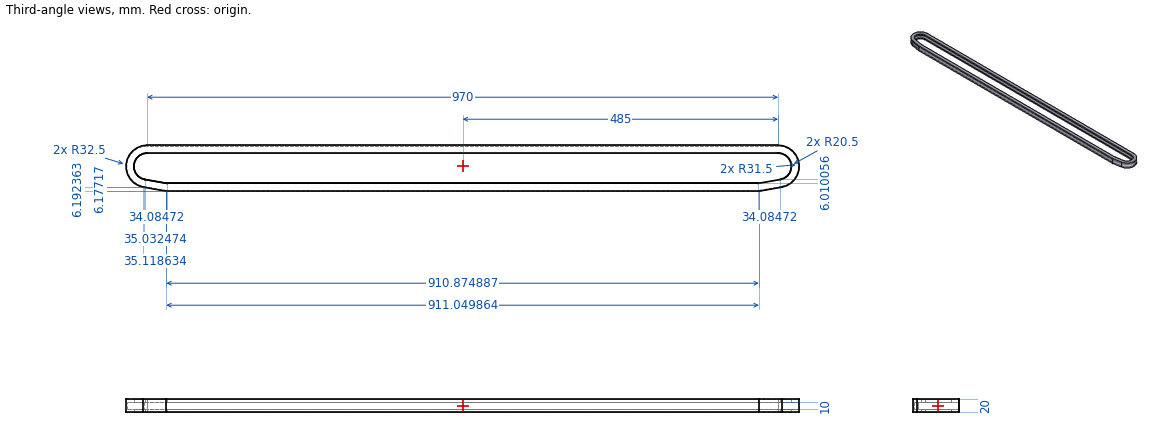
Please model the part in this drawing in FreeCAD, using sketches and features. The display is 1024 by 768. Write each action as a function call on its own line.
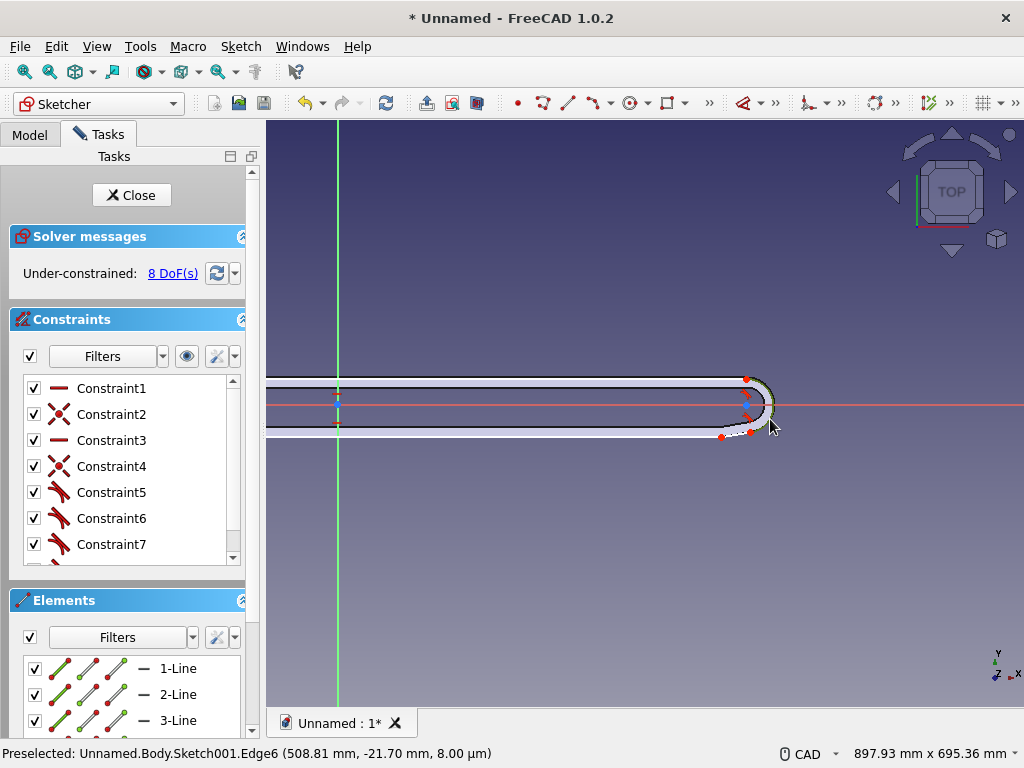
key(e)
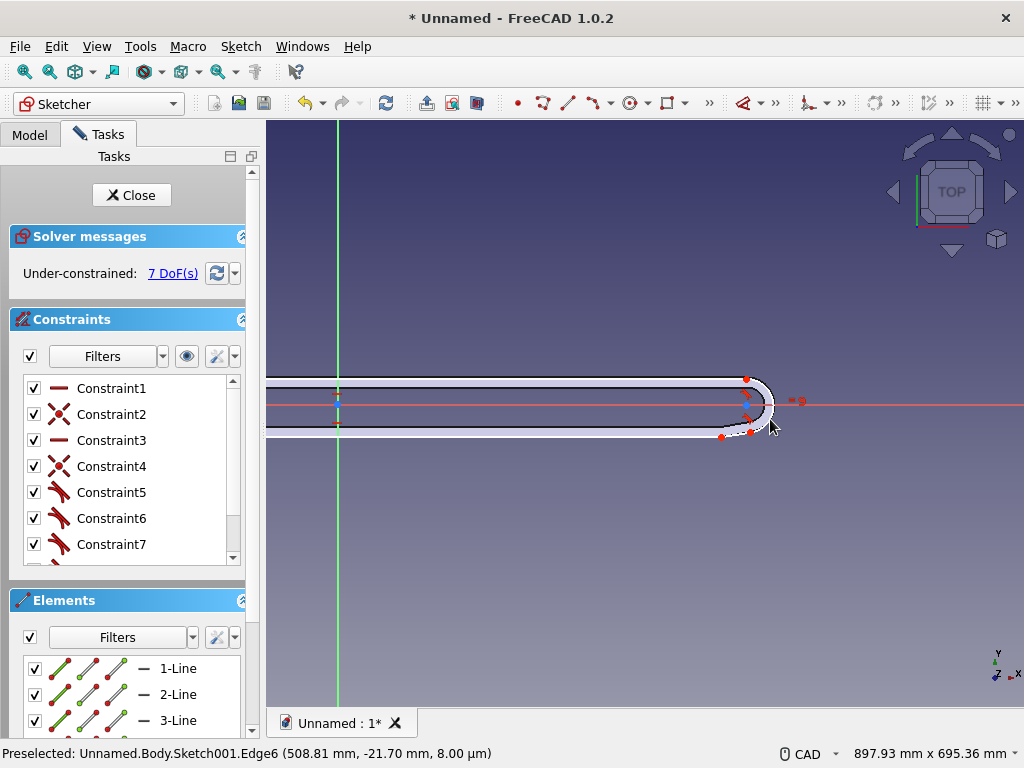
scroll(771, 419, down, 4)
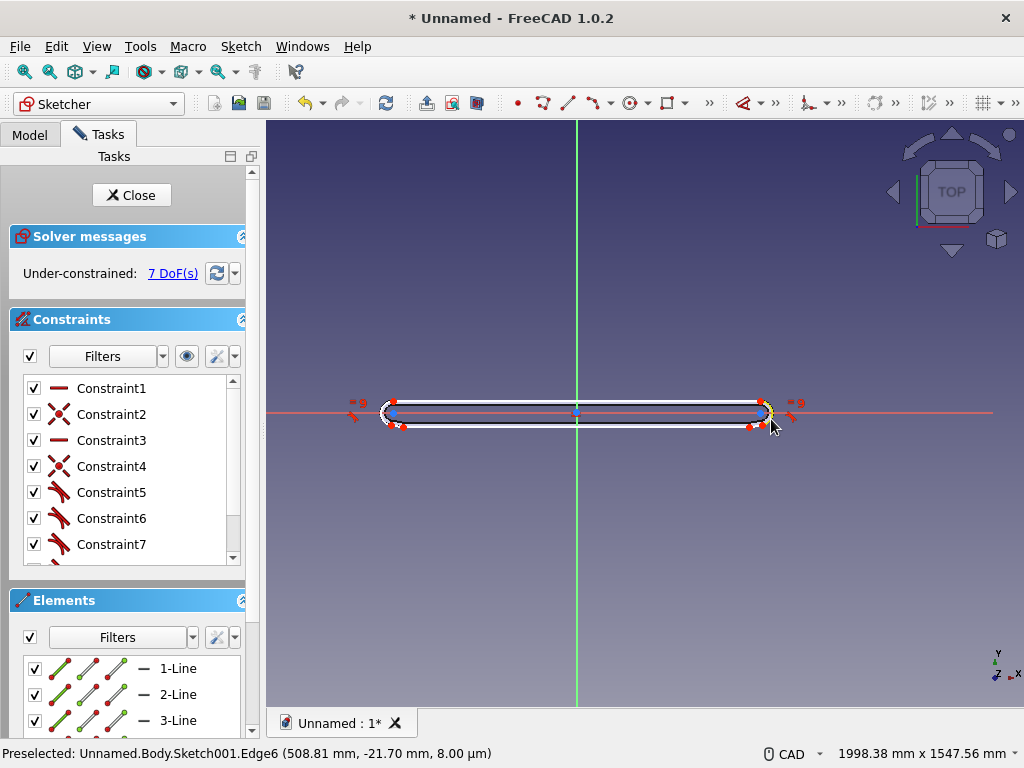
click(393, 413)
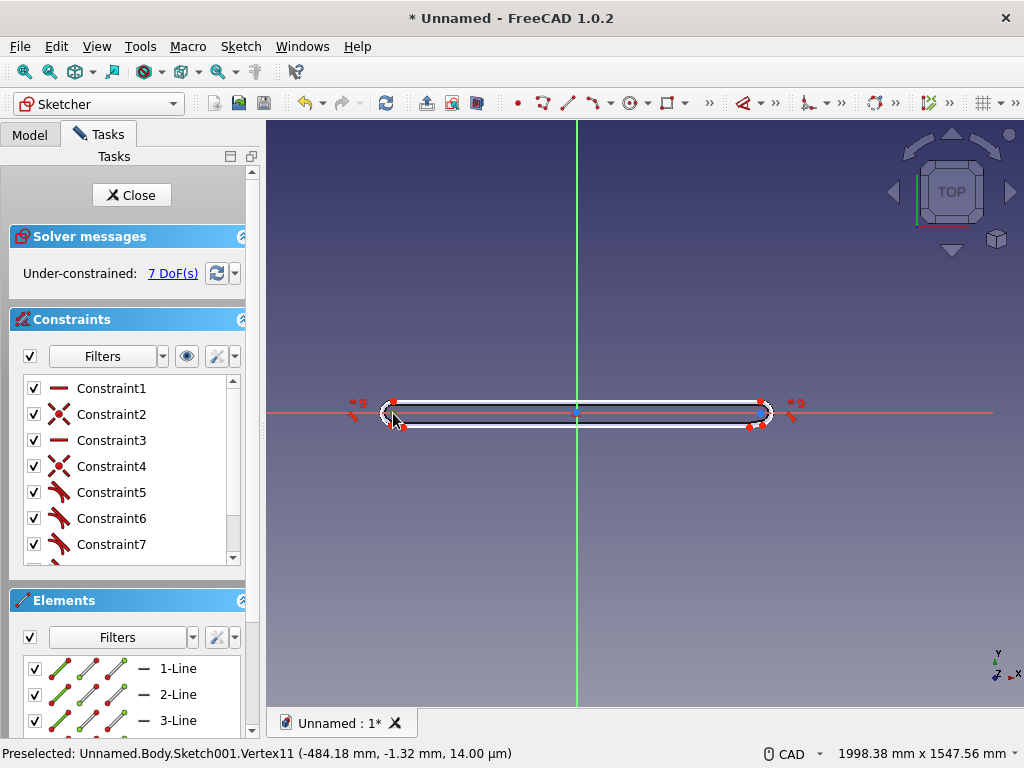
click(334, 413)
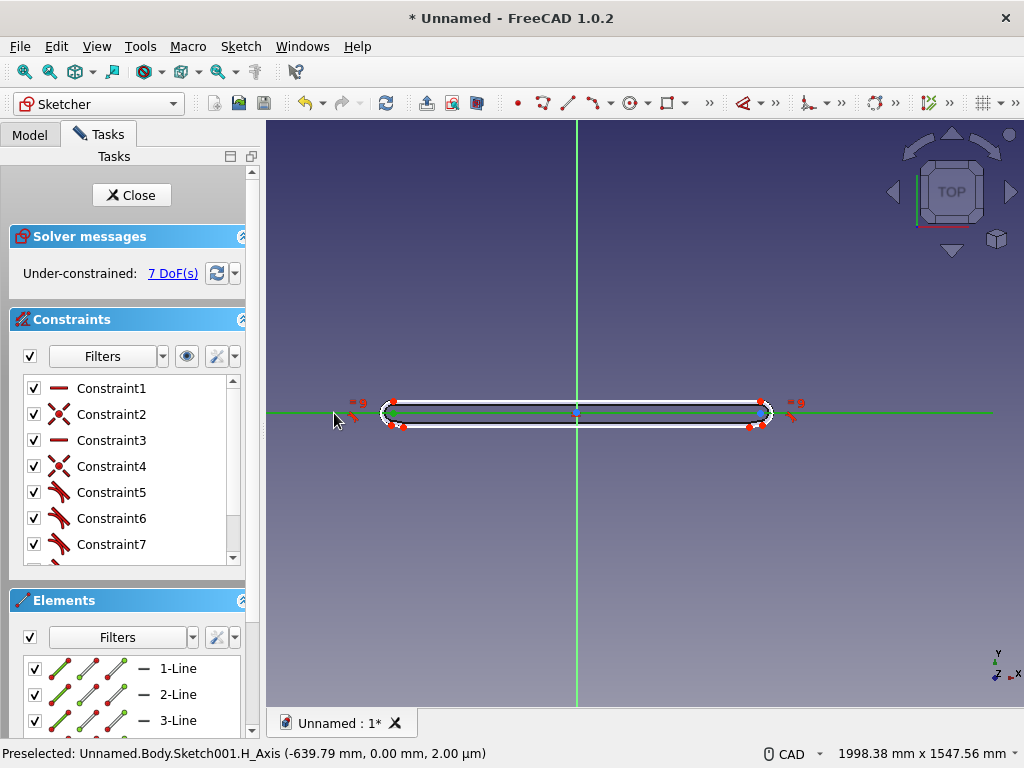
key(c)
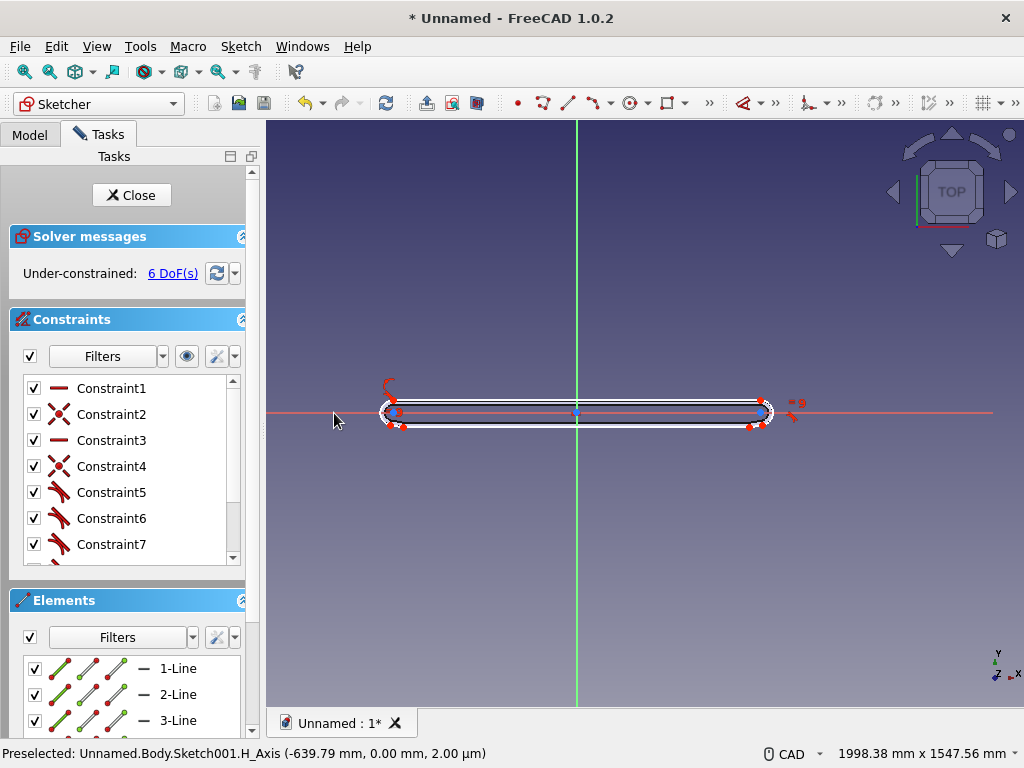
key(d)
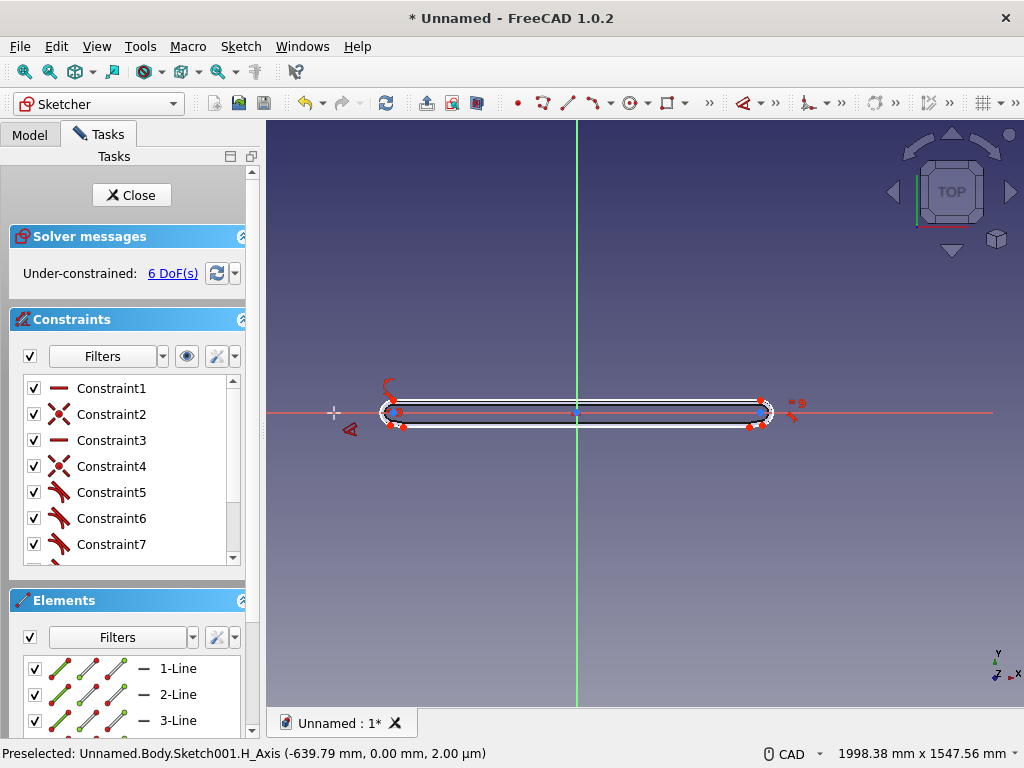
scroll(380, 412, up, 7)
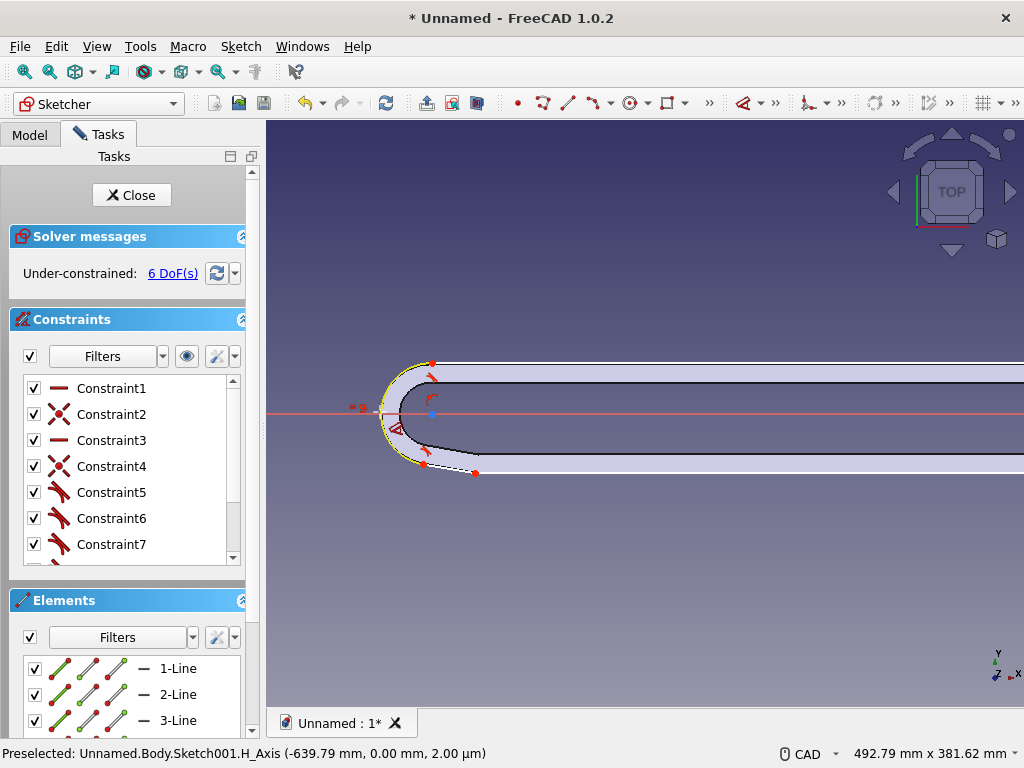
click(381, 410)
click(363, 368)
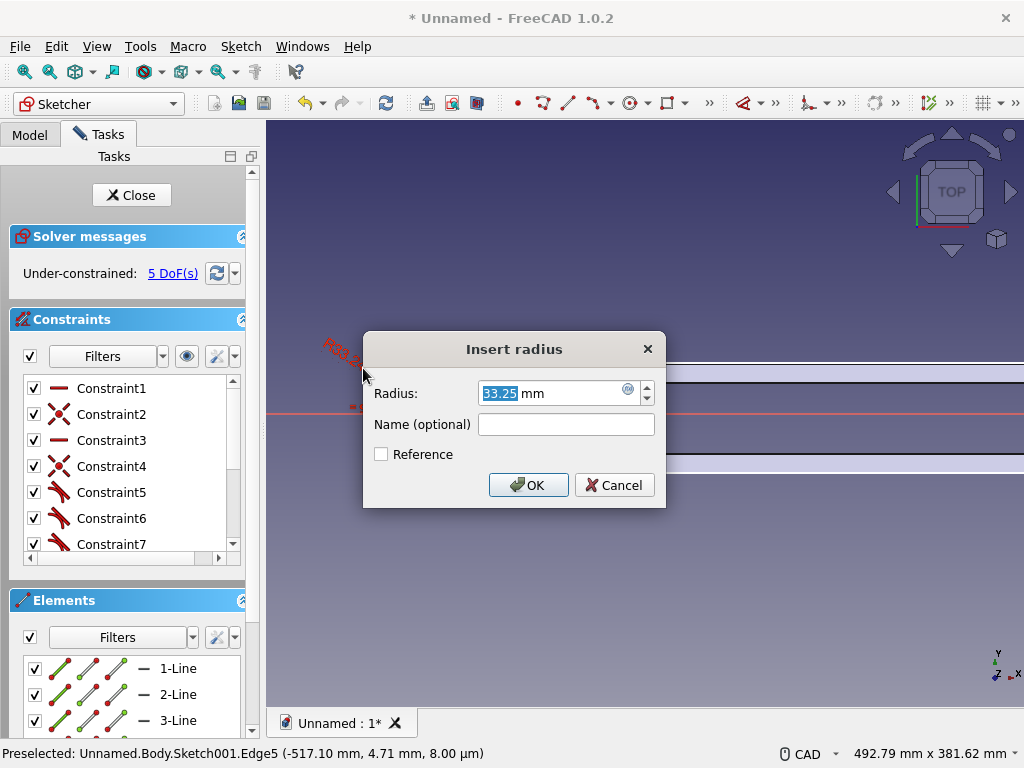
text(31.5)
key(Return)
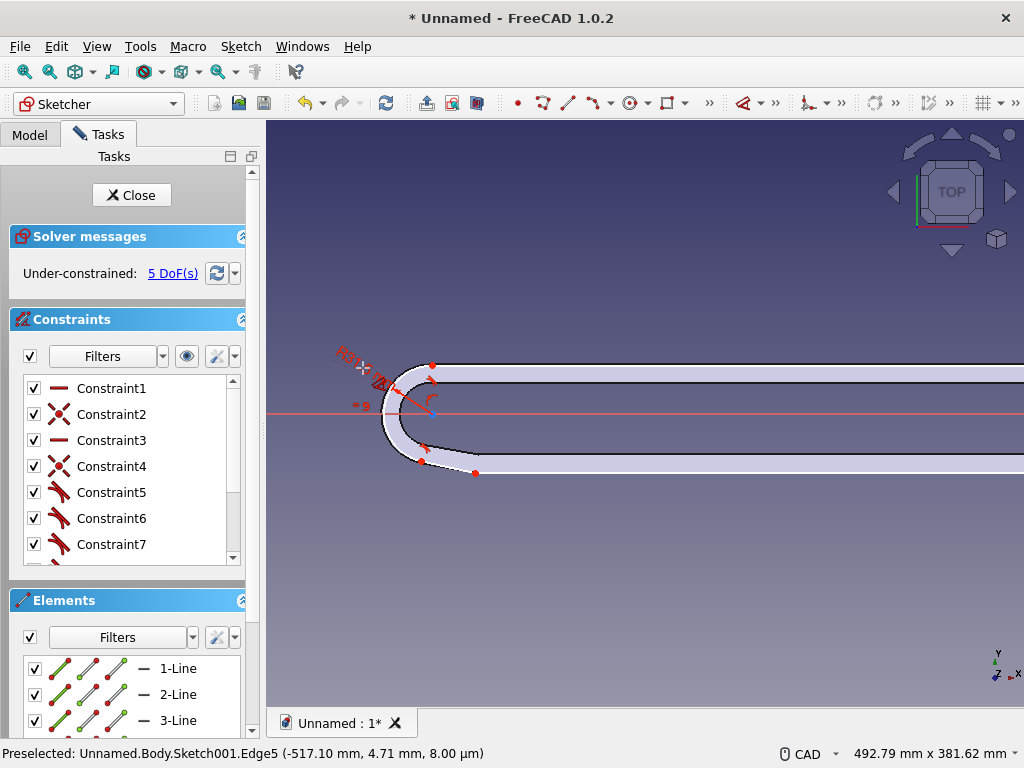
scroll(380, 412, down, 7)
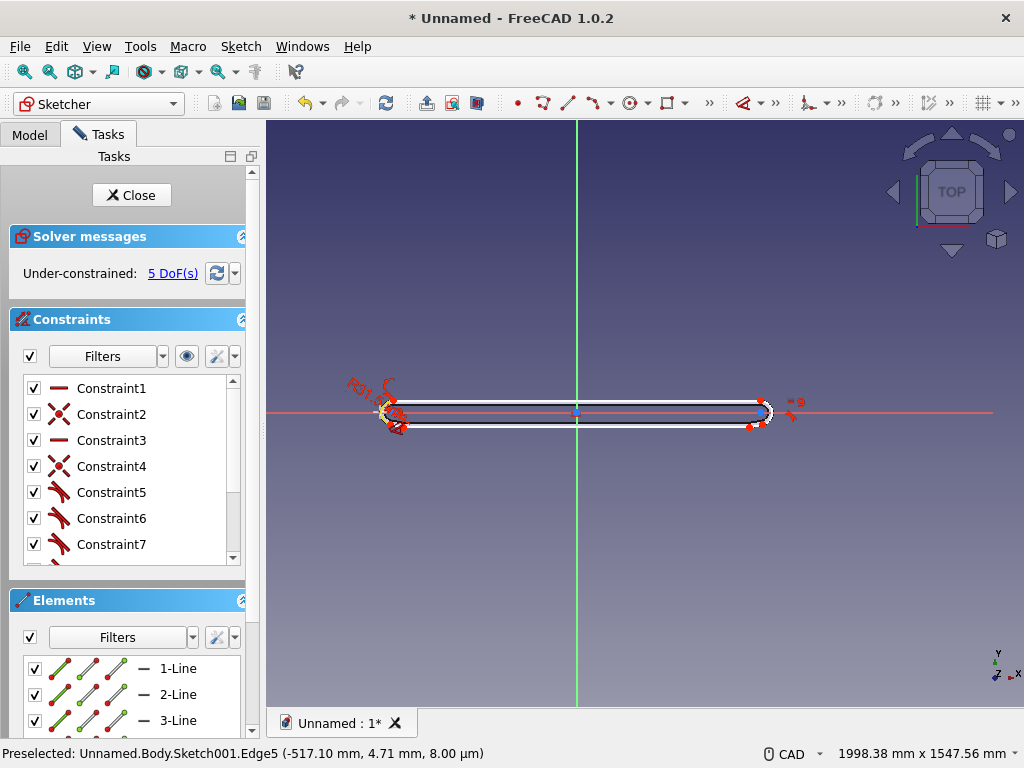
click(466, 401)
click(492, 367)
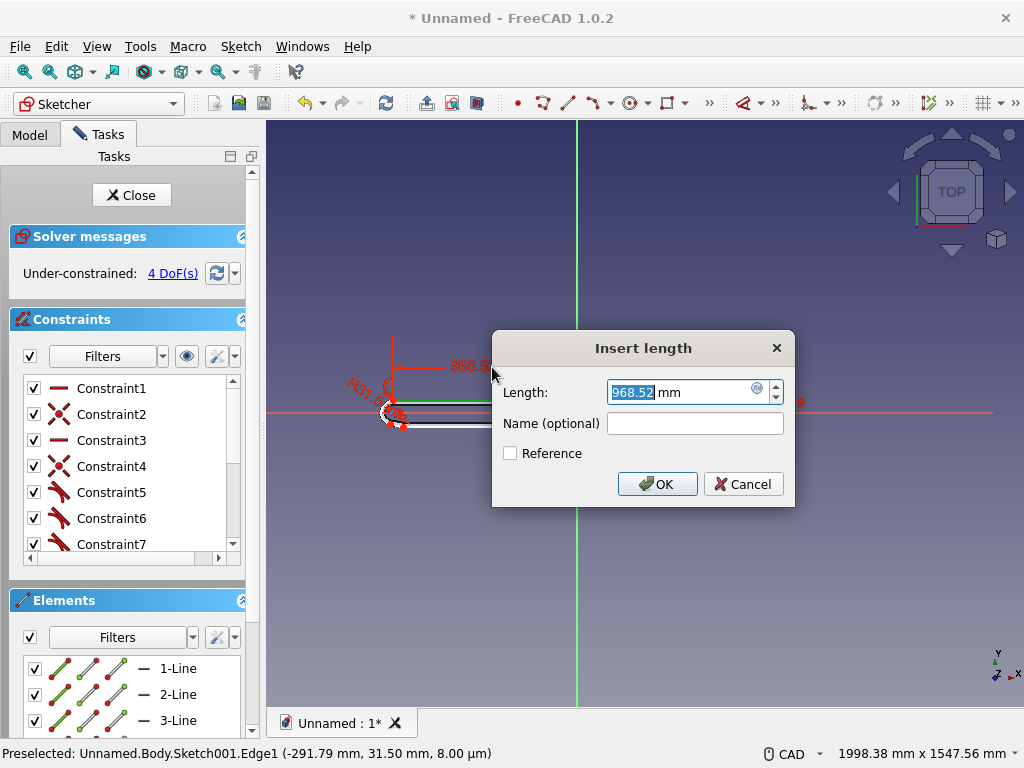
text(970)
key(Return)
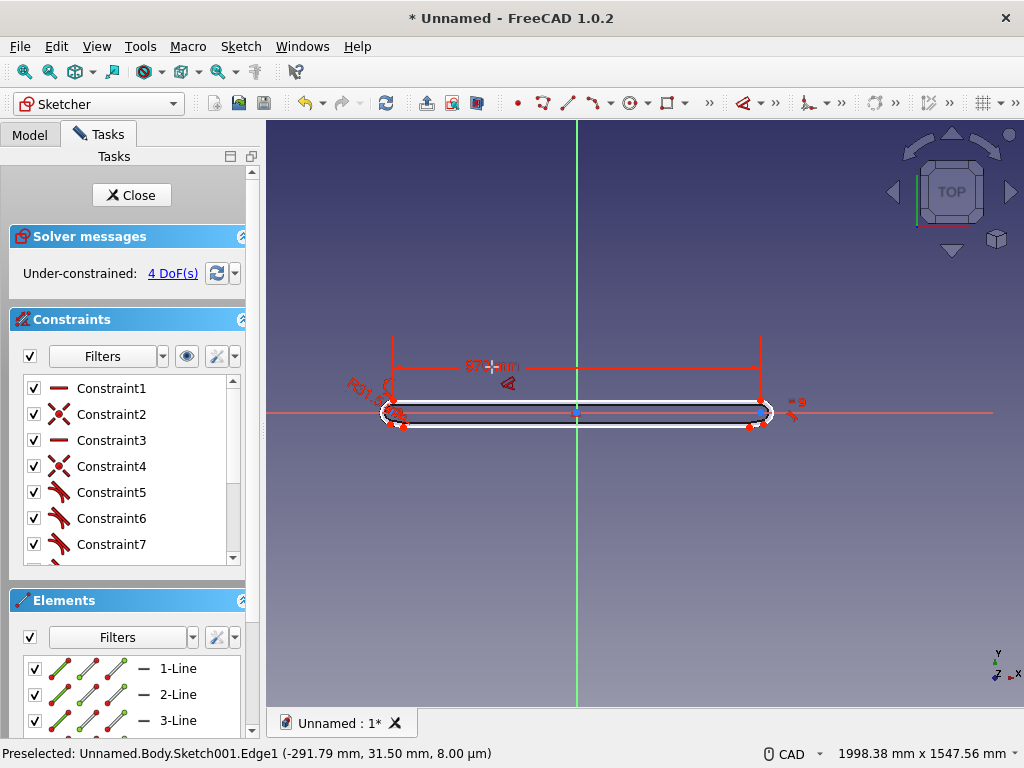
click(761, 401)
click(669, 367)